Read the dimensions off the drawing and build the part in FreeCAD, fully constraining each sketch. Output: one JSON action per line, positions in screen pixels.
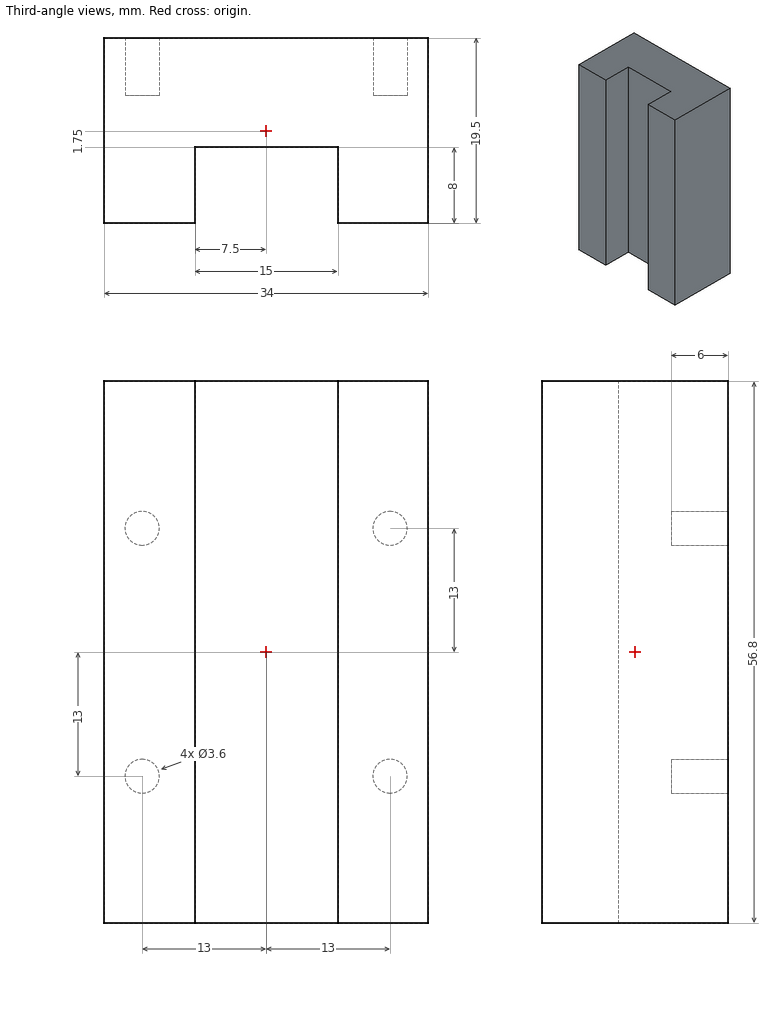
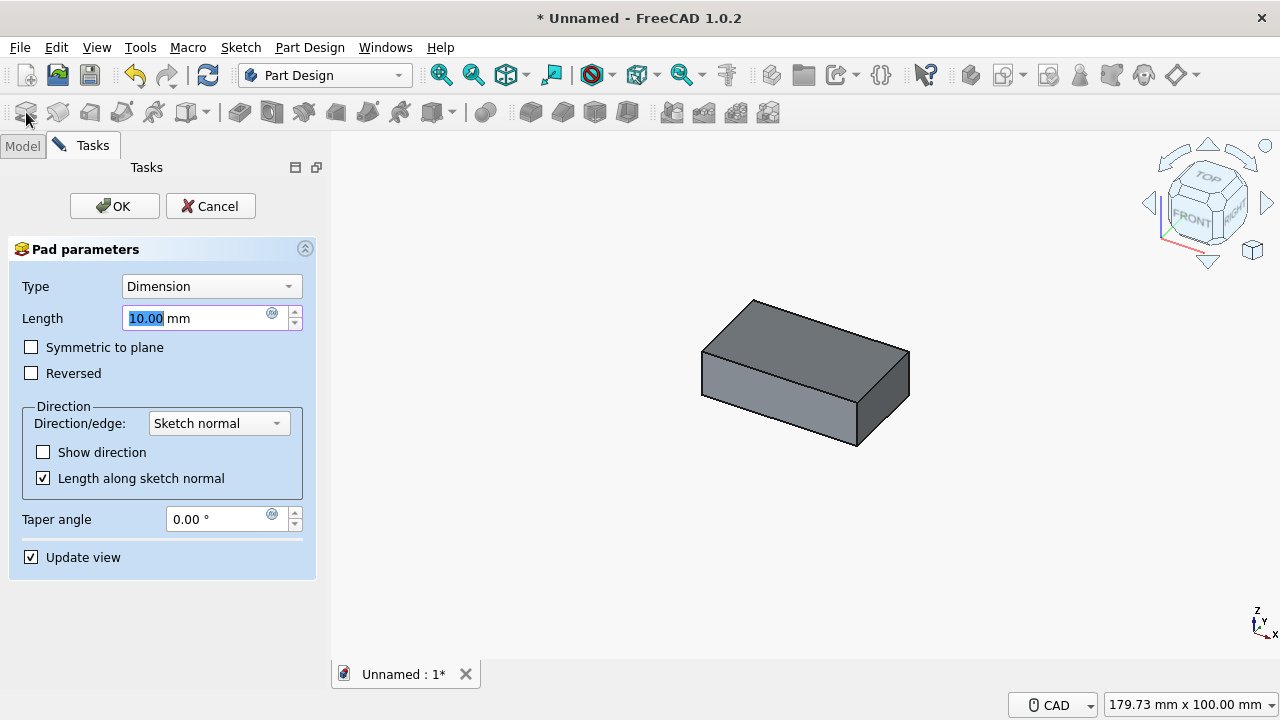
{"action": "type", "text": "56.8"}
{"action": "key", "text": "Tab"}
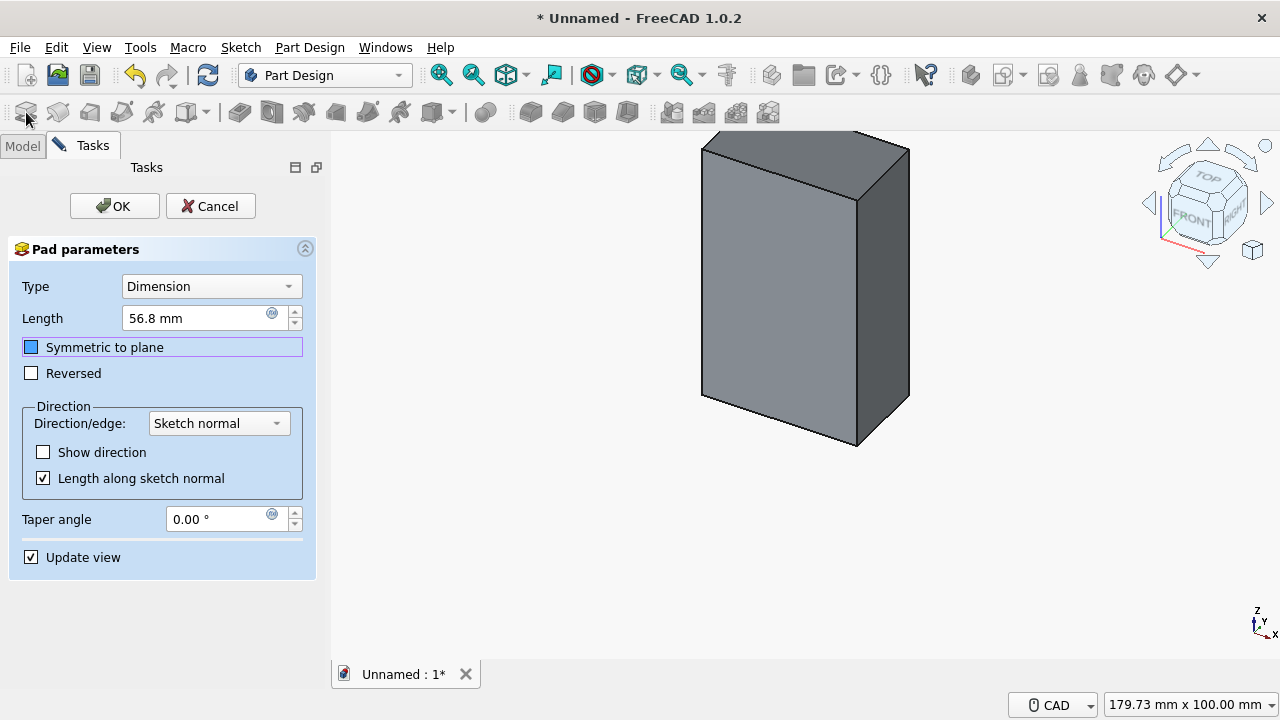
{"action": "left_click", "coordinate": [30, 347]}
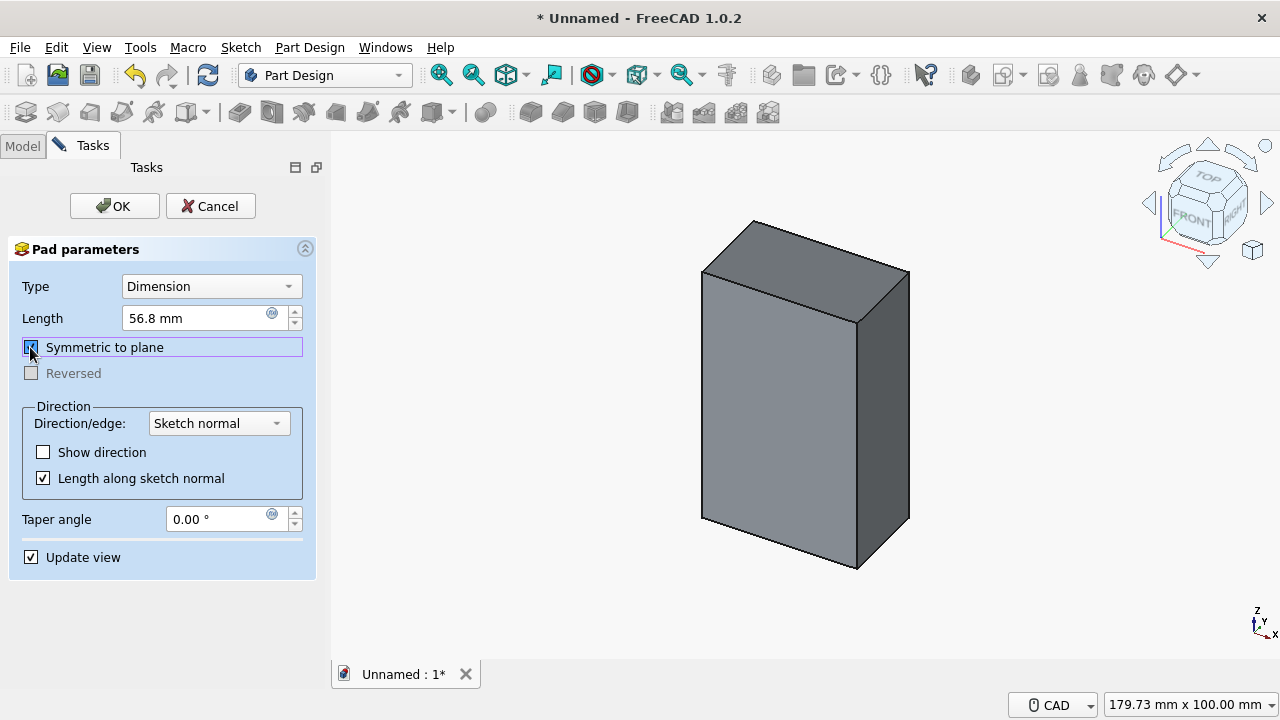
{"action": "left_click", "coordinate": [115, 206]}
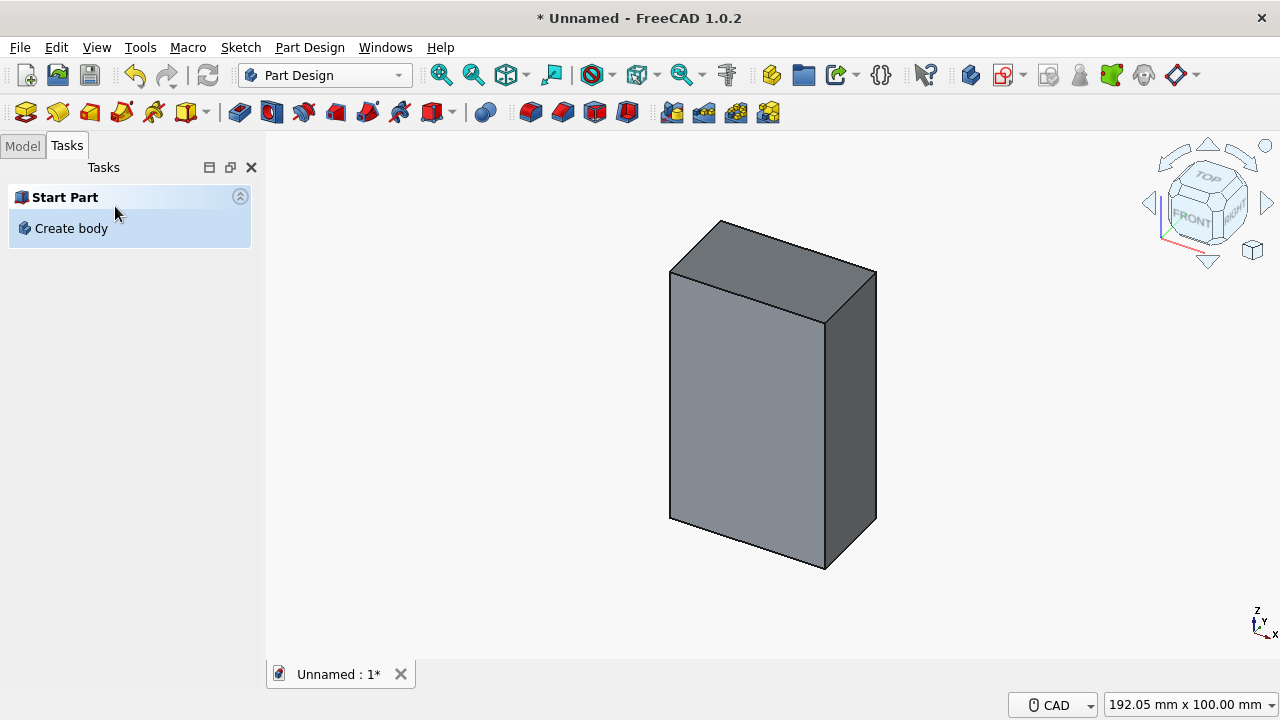
{"action": "left_click", "coordinate": [1004, 76]}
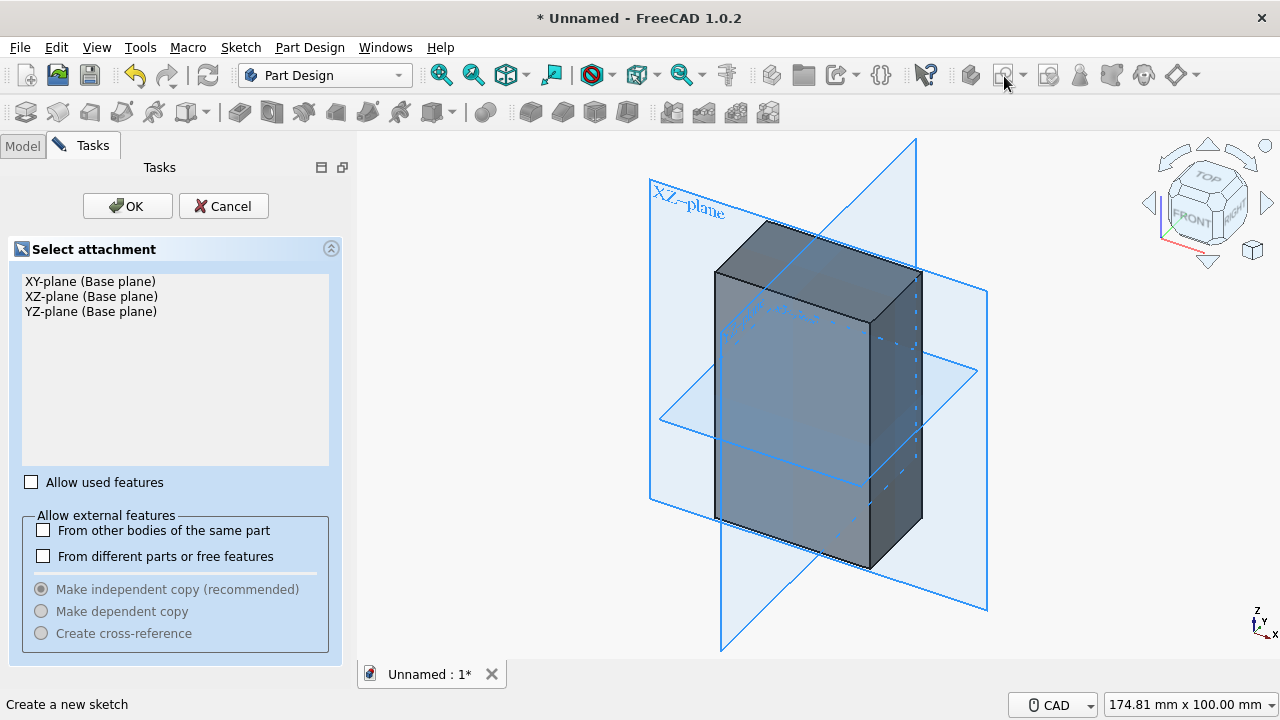
{"action": "left_click", "coordinate": [82, 282]}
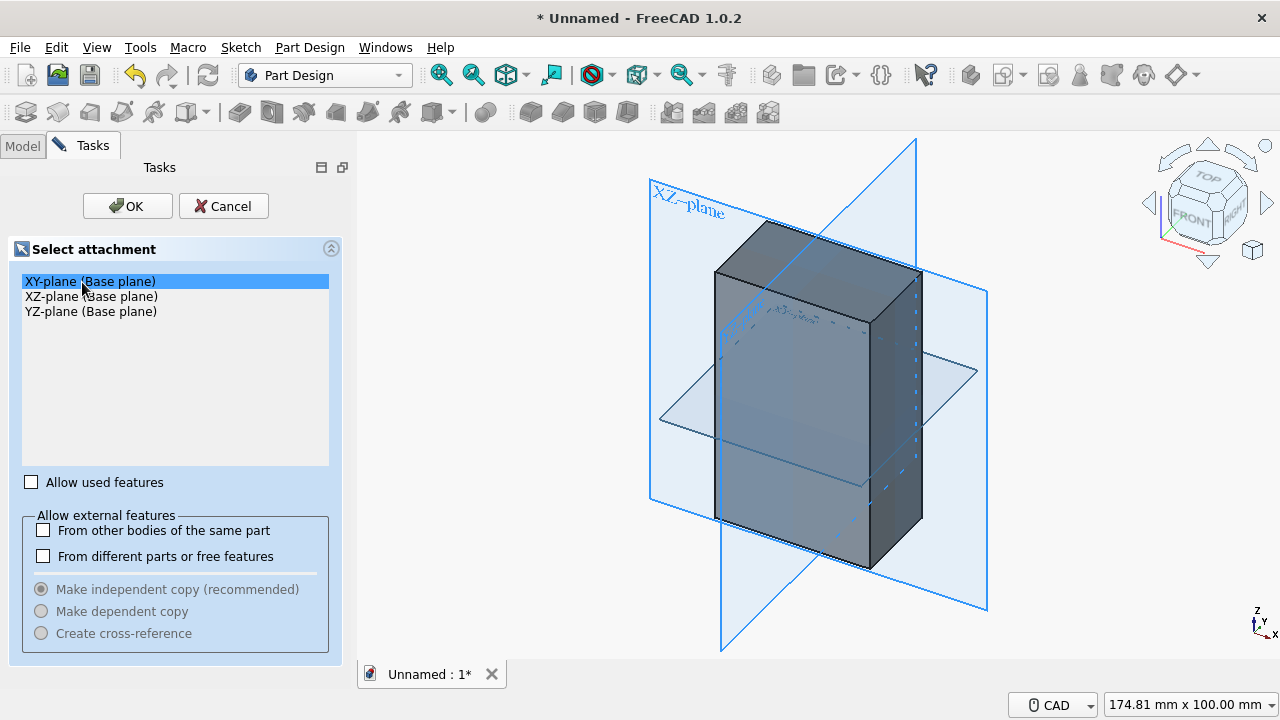
{"action": "left_click", "coordinate": [128, 206]}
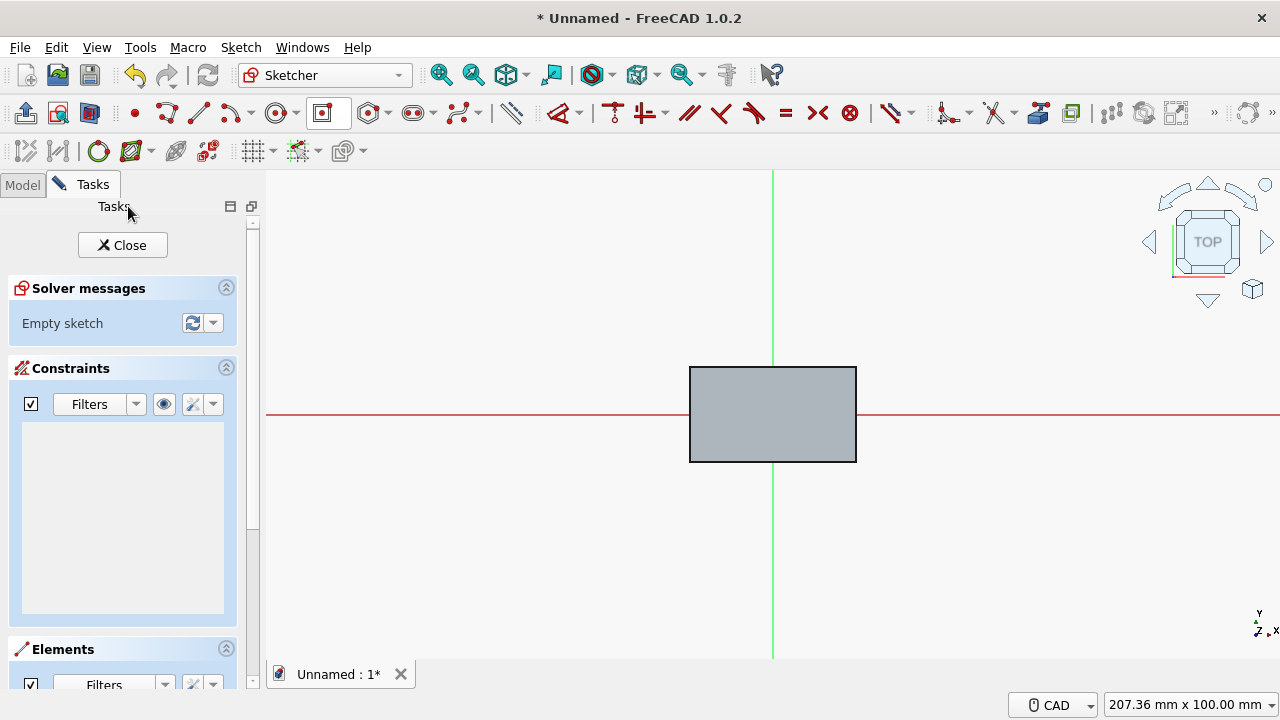
{"action": "left_click", "coordinate": [90, 114]}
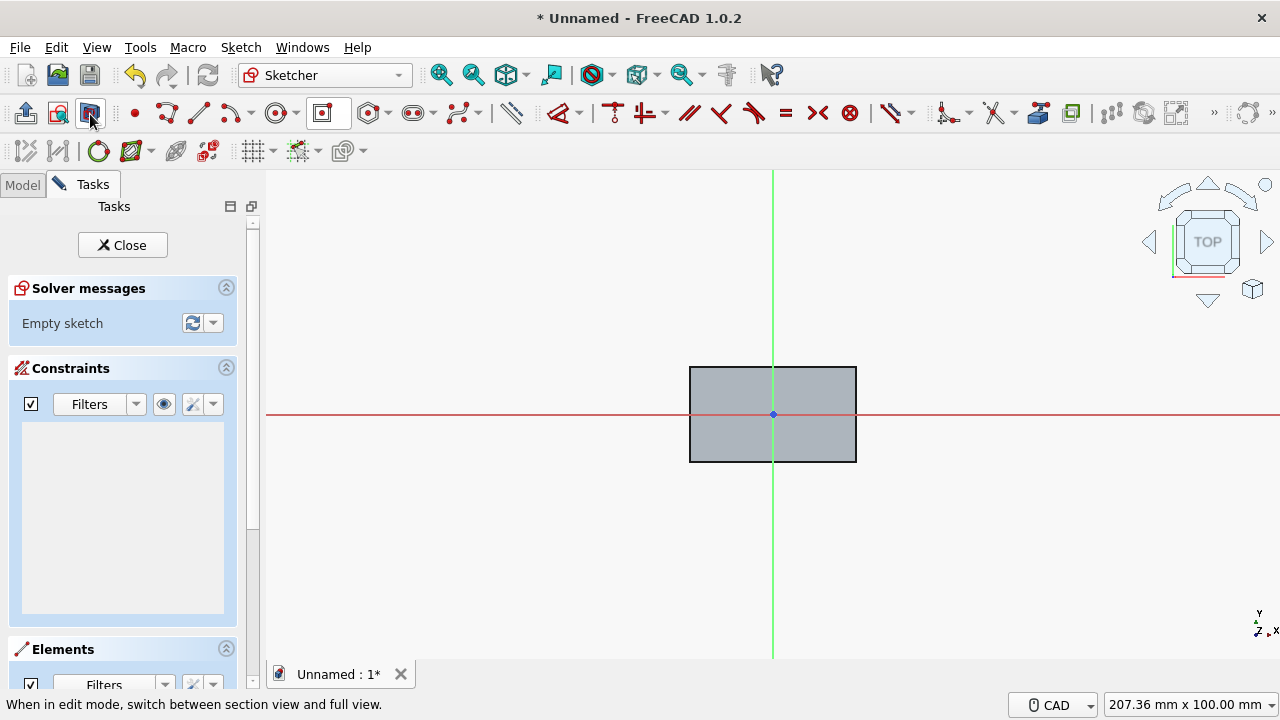
{"action": "scroll", "coordinate": [787, 443], "scroll_direction": "up", "scroll_amount": 9}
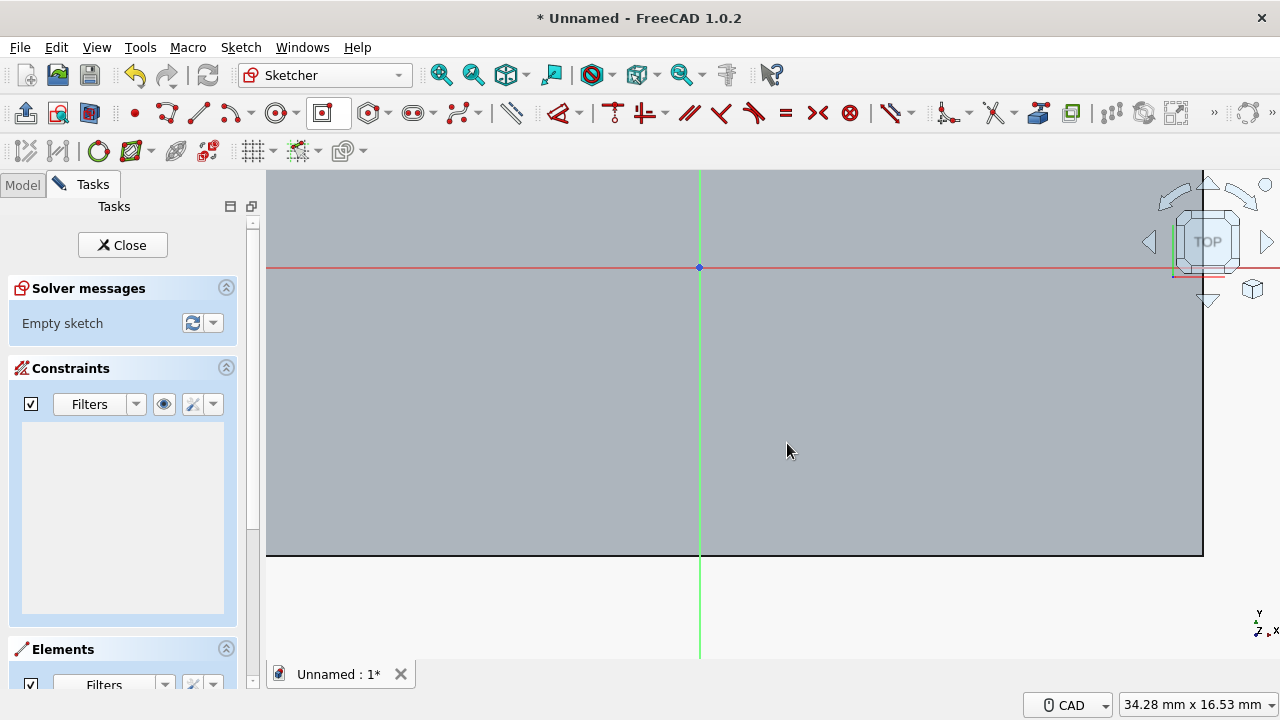
{"action": "key", "text": "g r"}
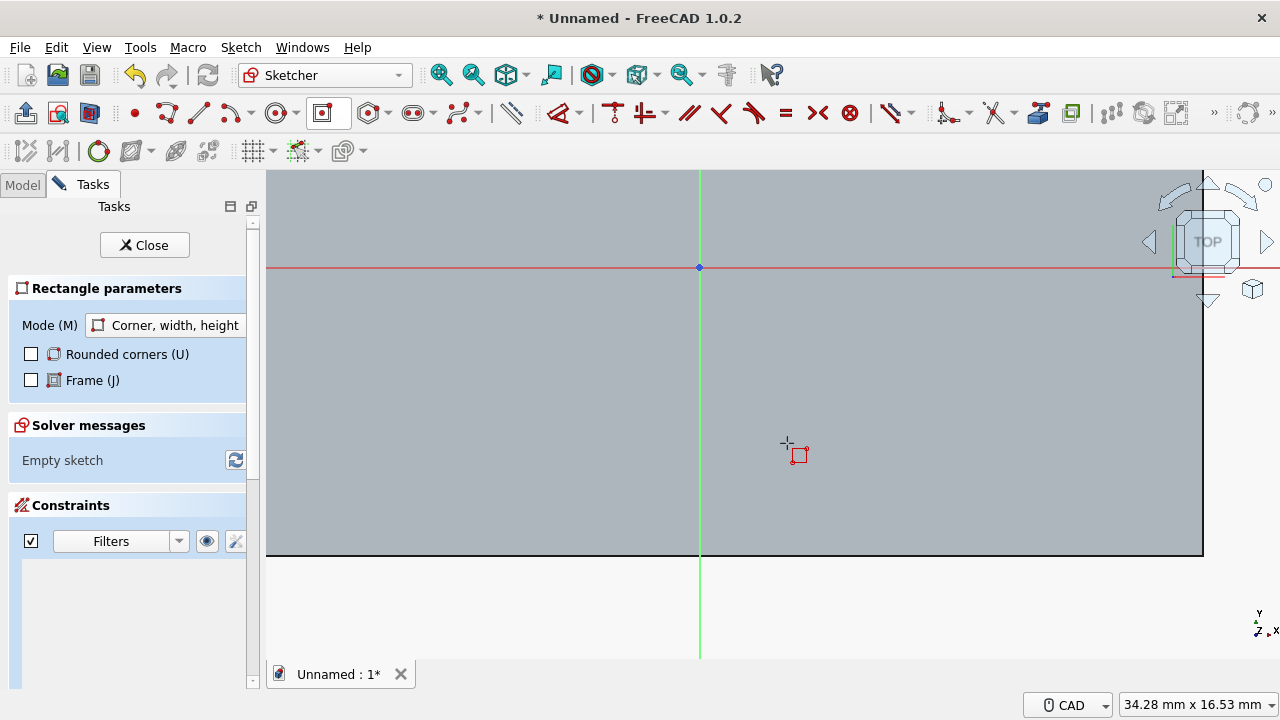
{"action": "left_click", "coordinate": [478, 320]}
{"action": "mouse_move", "coordinate": [922, 556]}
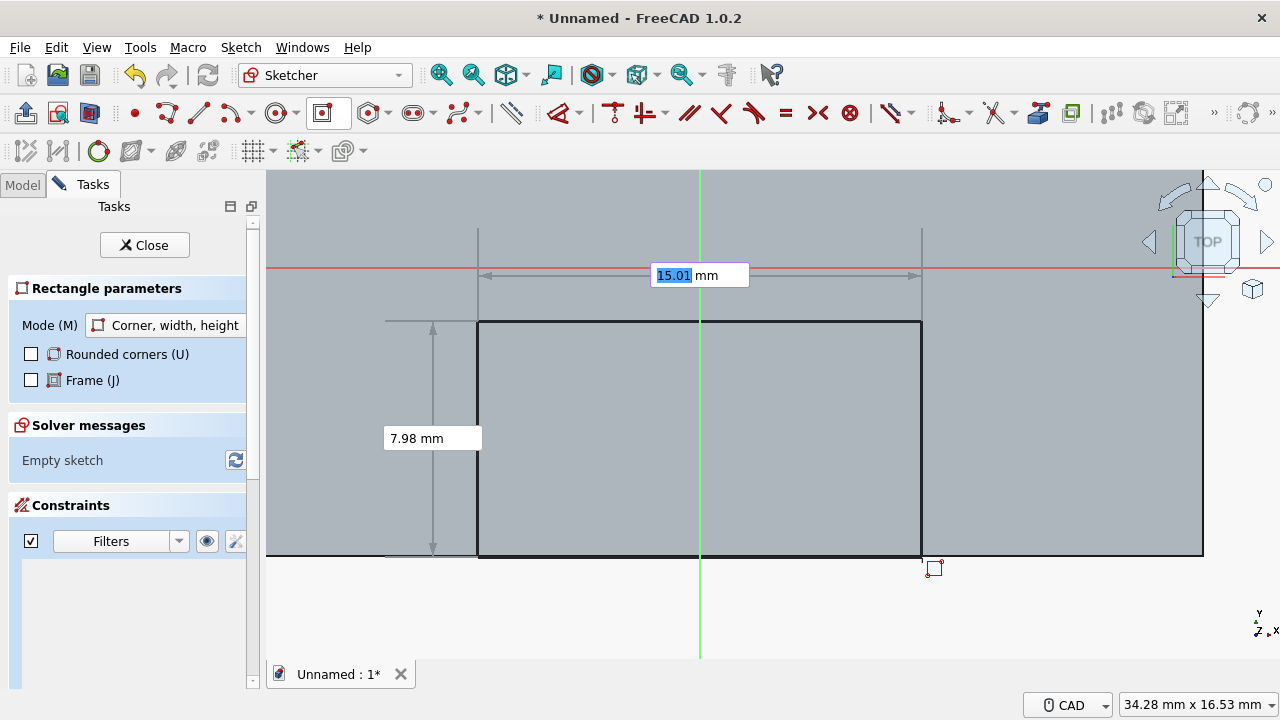
{"action": "type", "text": "15"}
{"action": "key", "text": "Tab"}
{"action": "type", "text": "8"}
{"action": "key", "text": "Return"}
{"action": "key", "text": "Escape"}